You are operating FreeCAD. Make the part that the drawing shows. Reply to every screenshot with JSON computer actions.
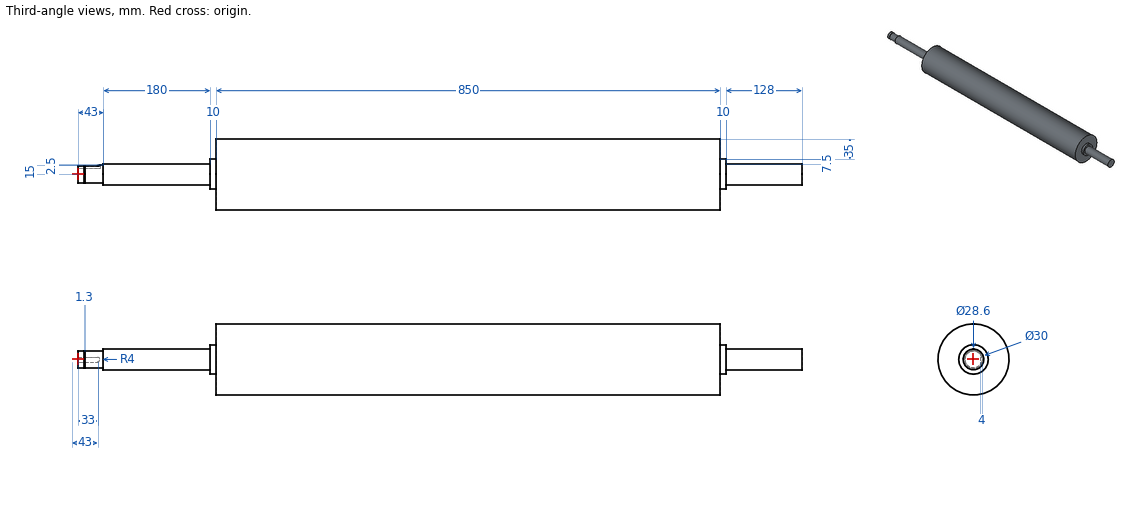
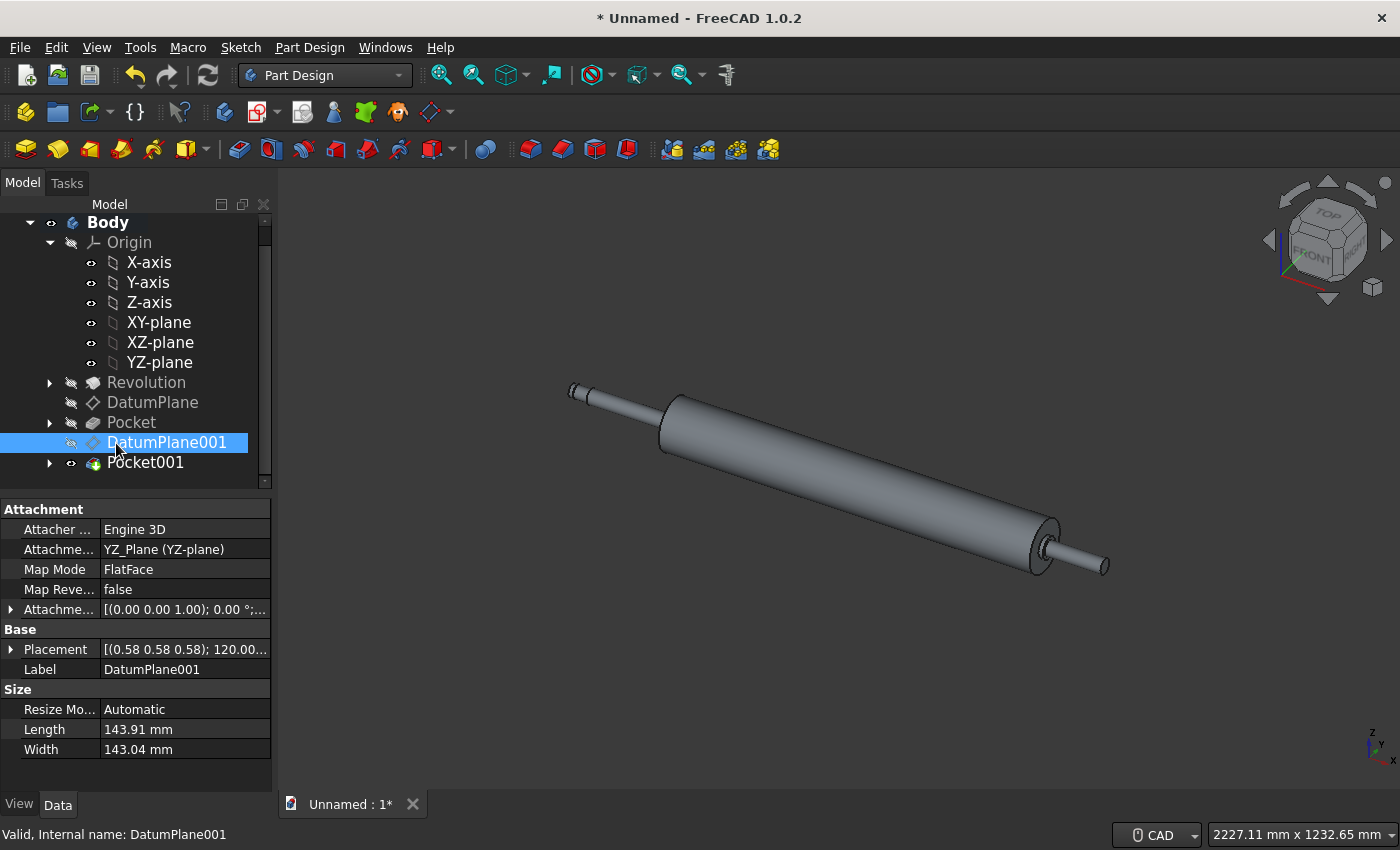
{"action": "key", "text": "0"}